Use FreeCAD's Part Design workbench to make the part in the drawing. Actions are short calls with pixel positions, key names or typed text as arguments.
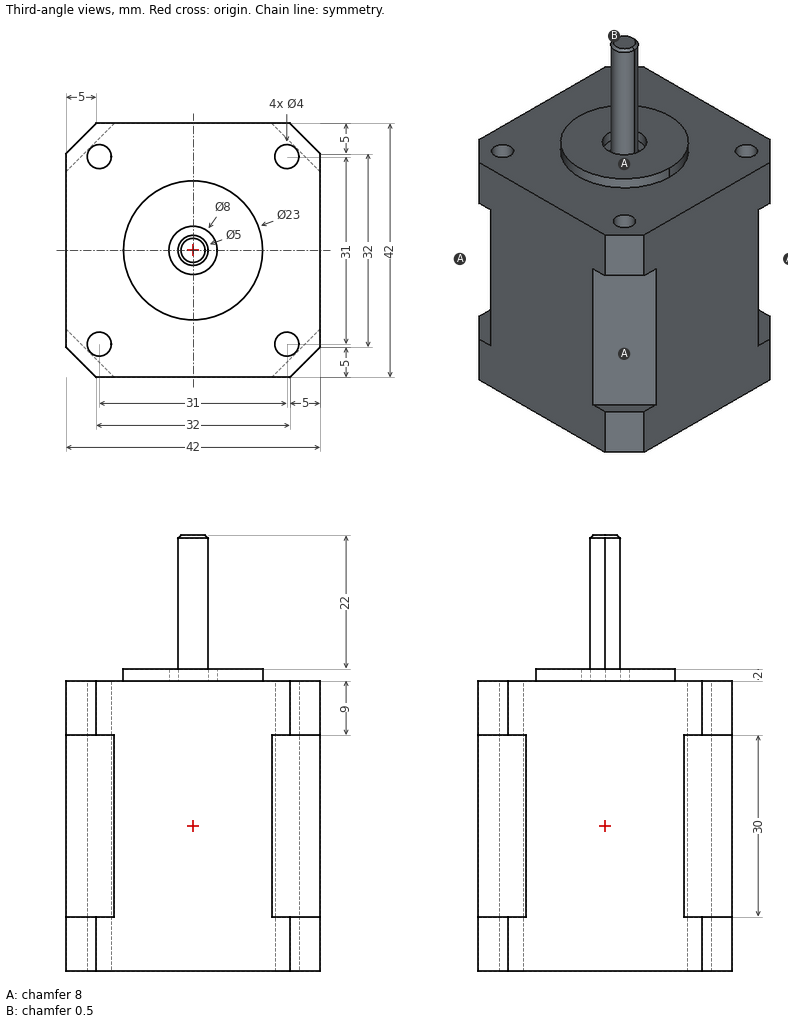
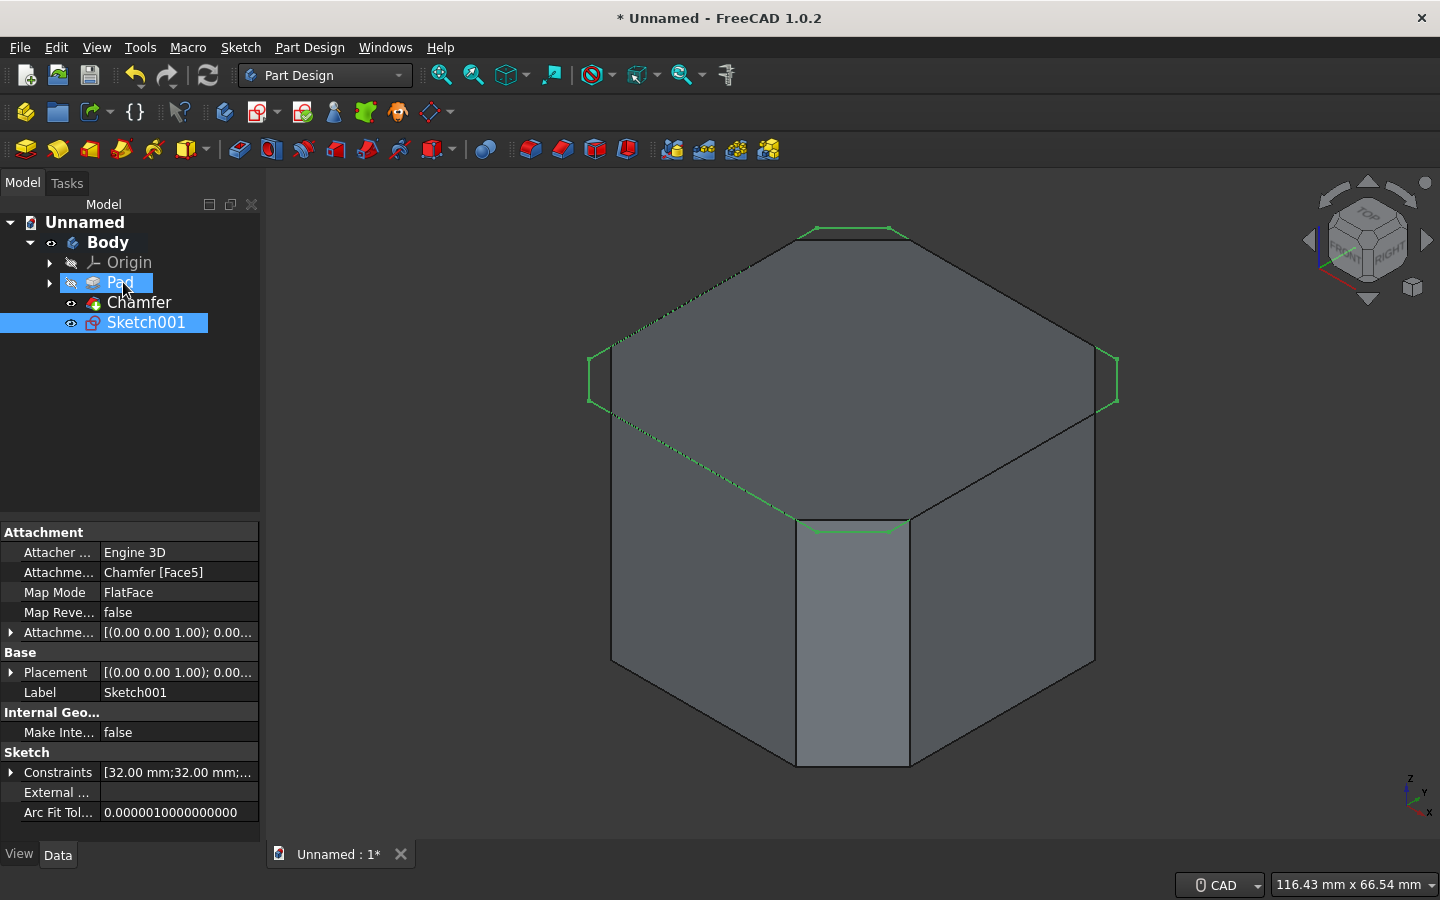
click(26, 150)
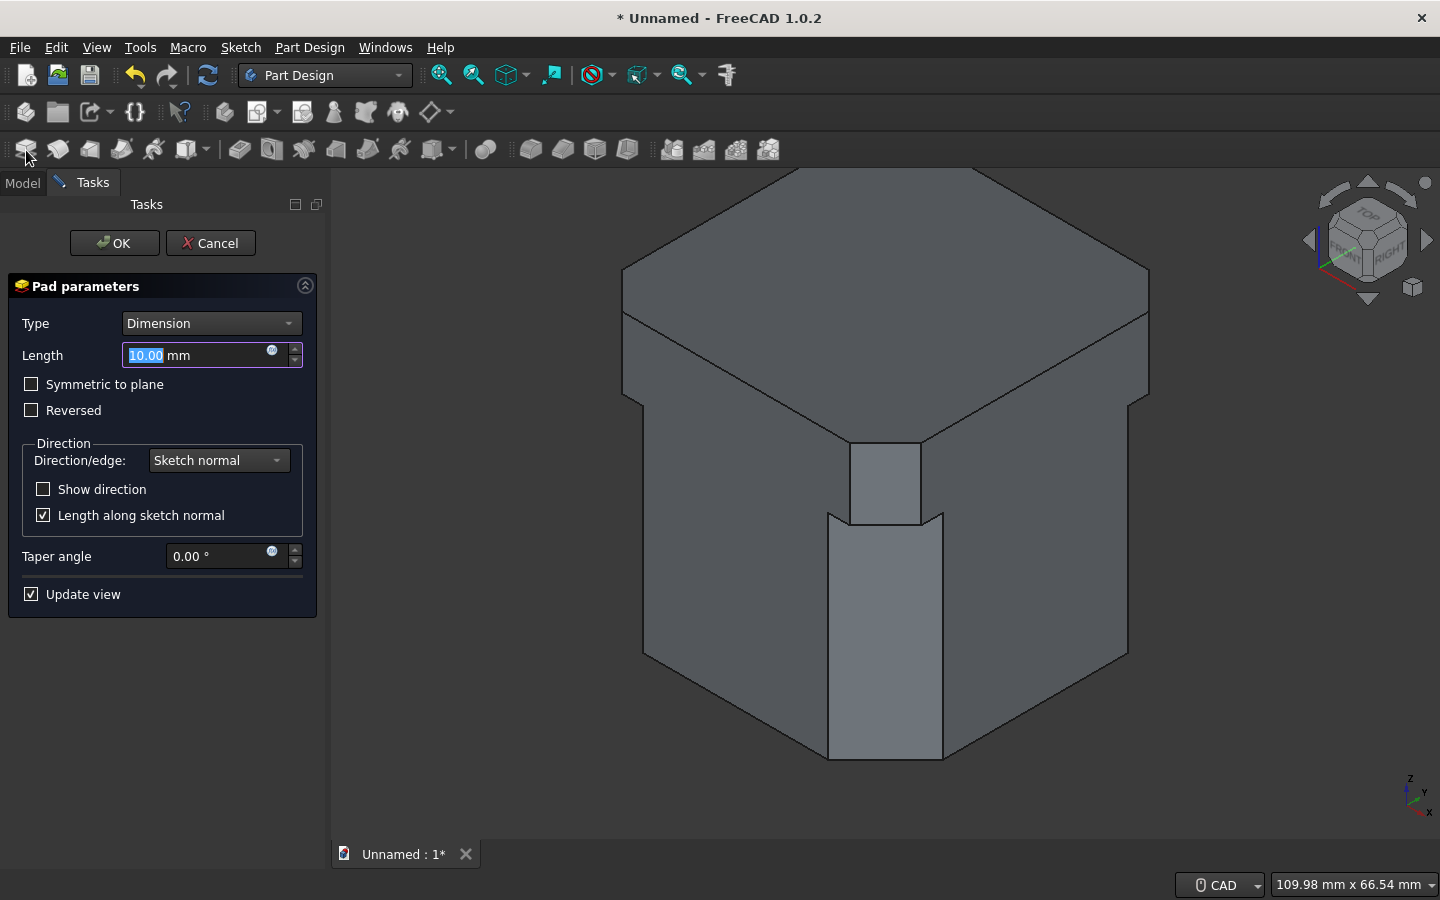
text(9)
key(Tab)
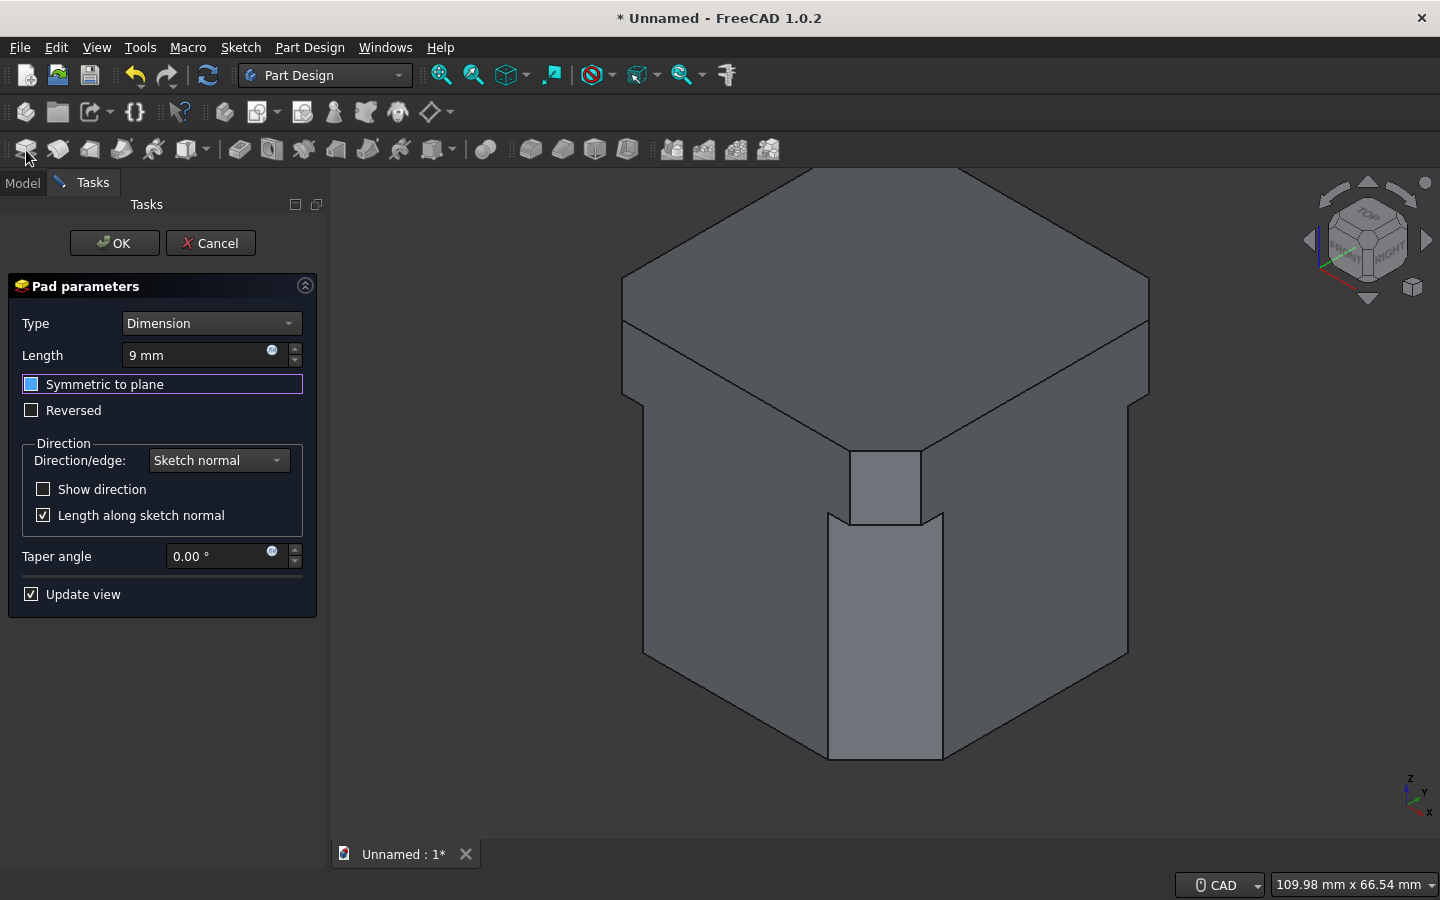
click(115, 243)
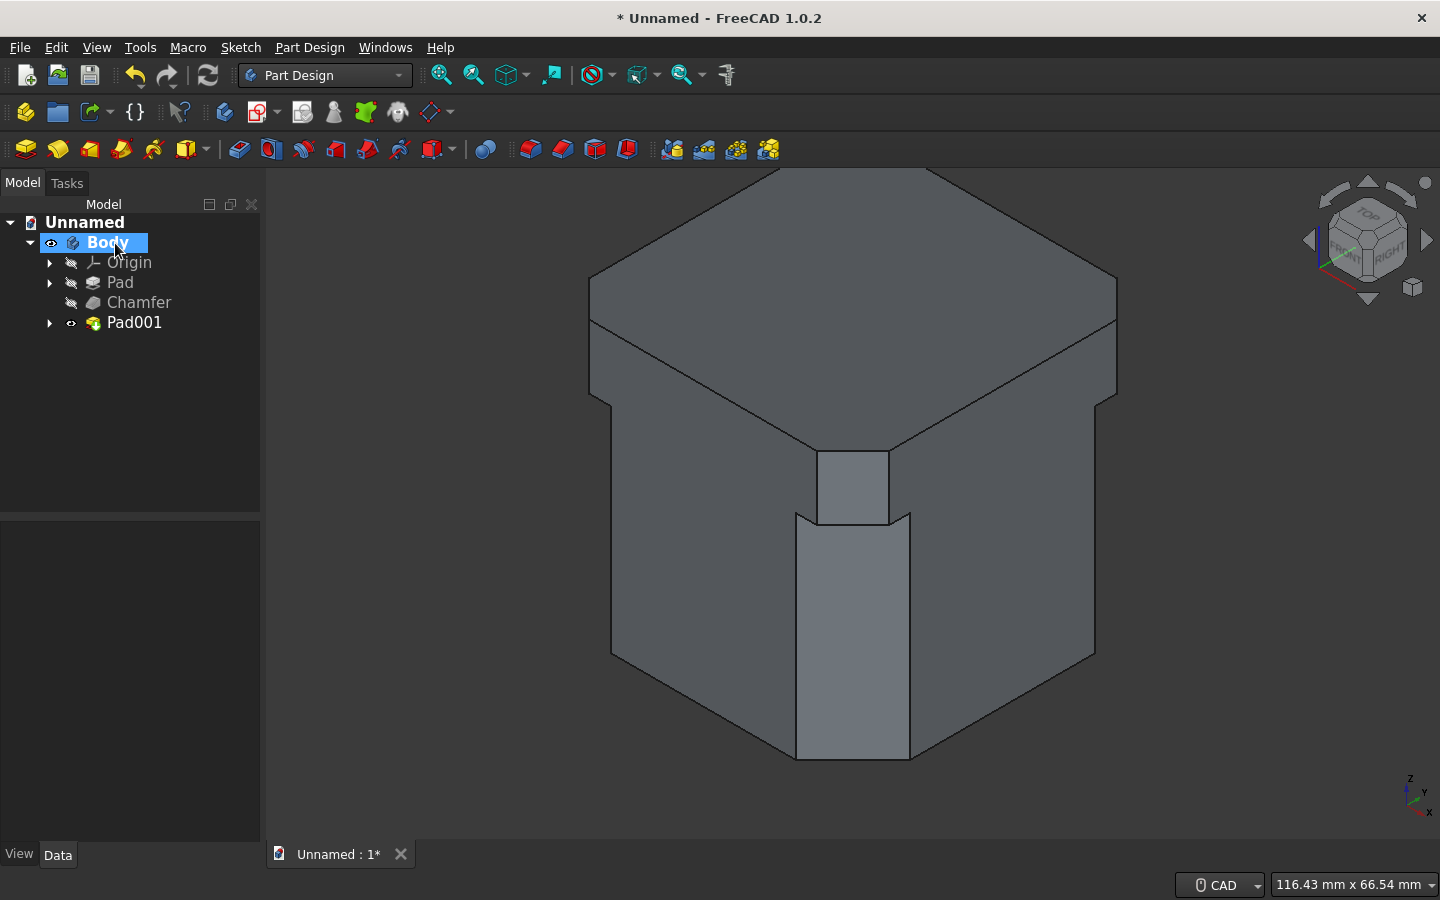
click(442, 76)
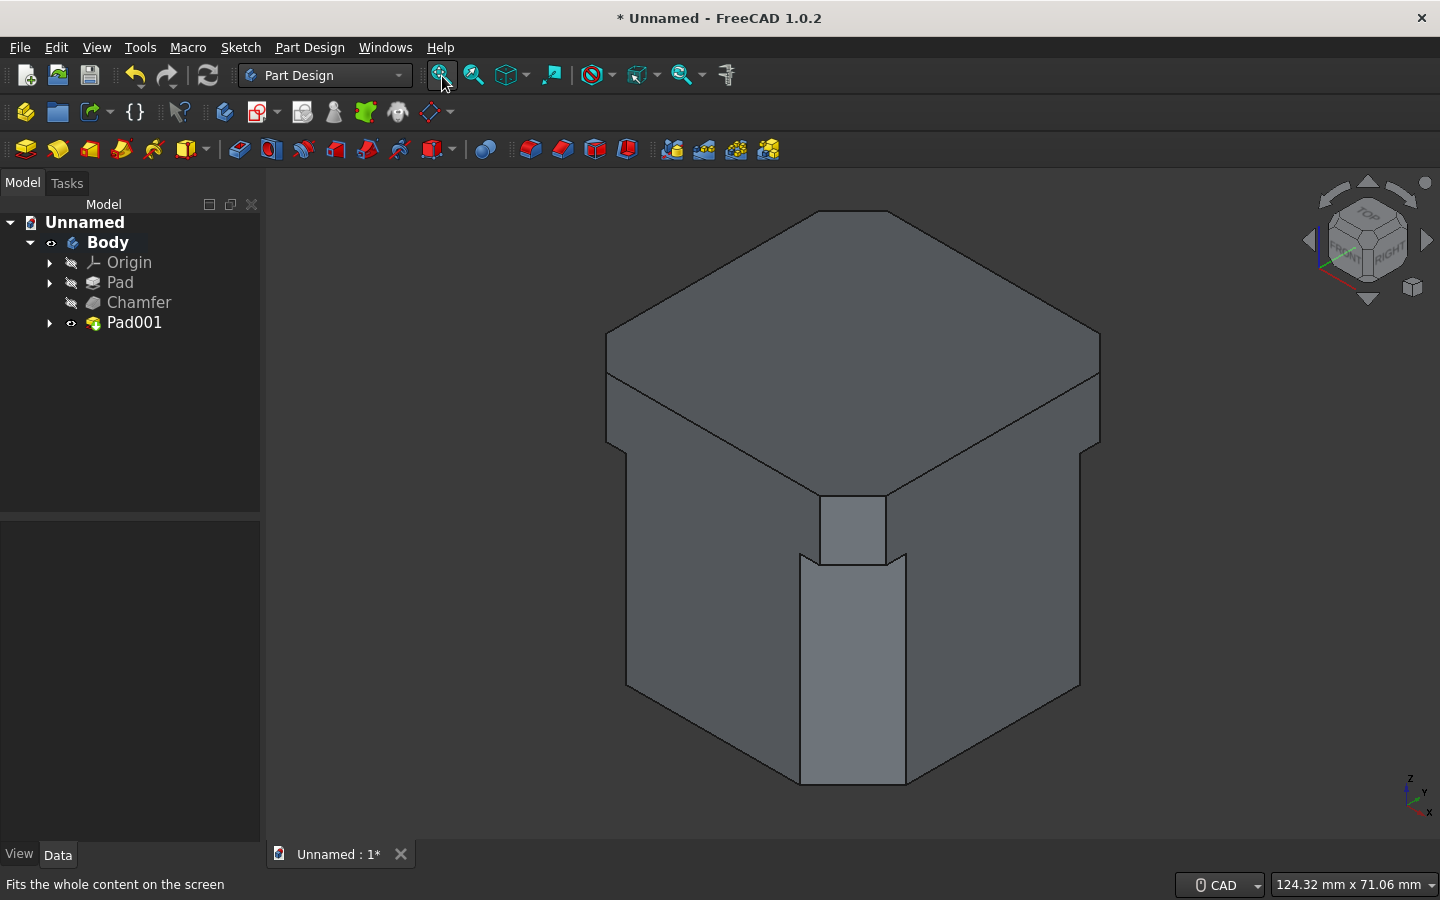
click(116, 323)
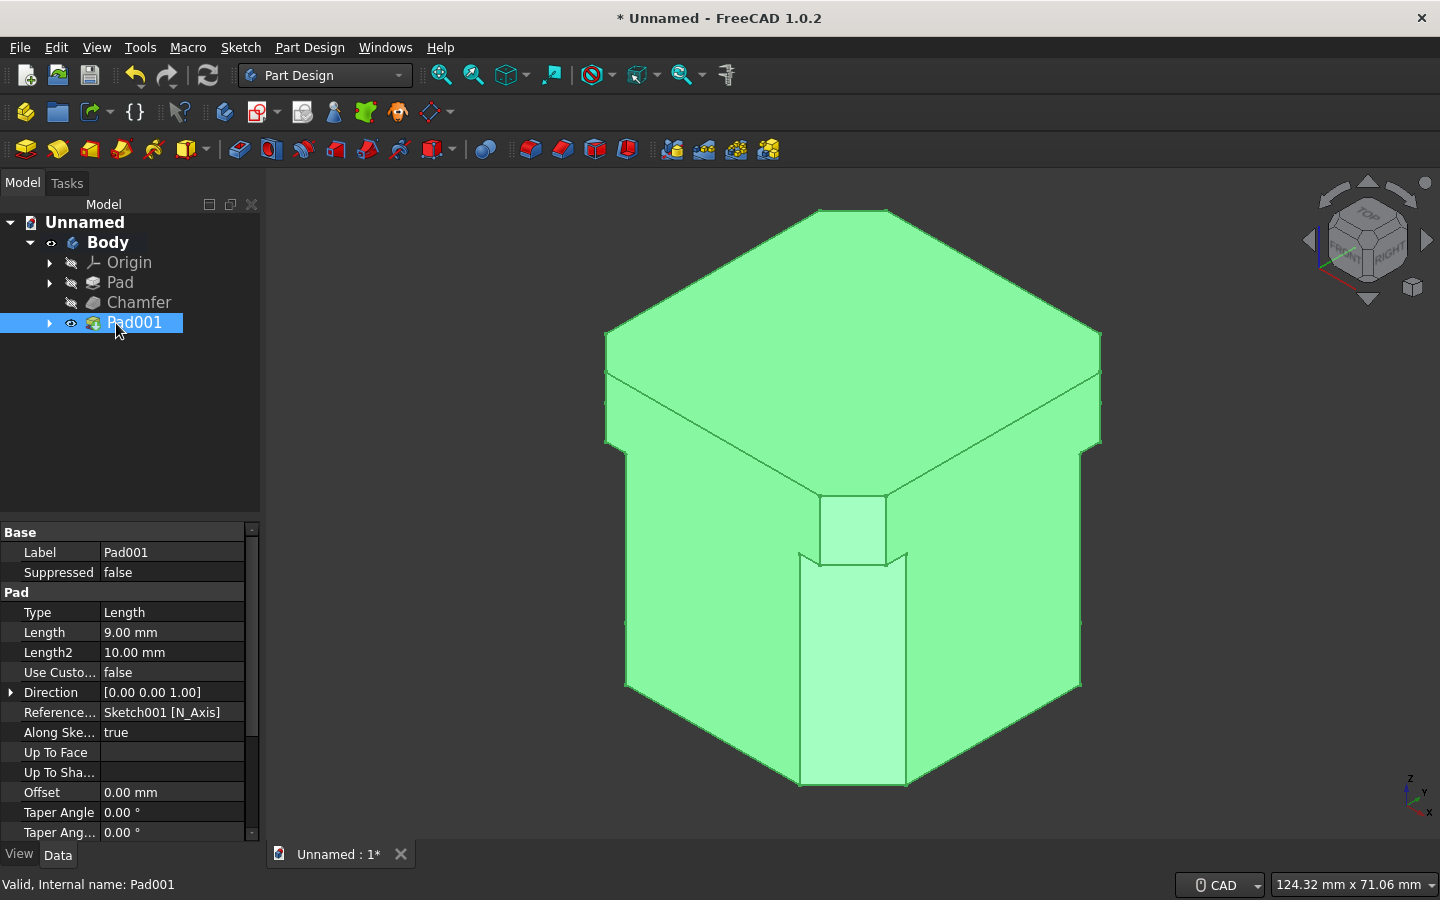
click(672, 150)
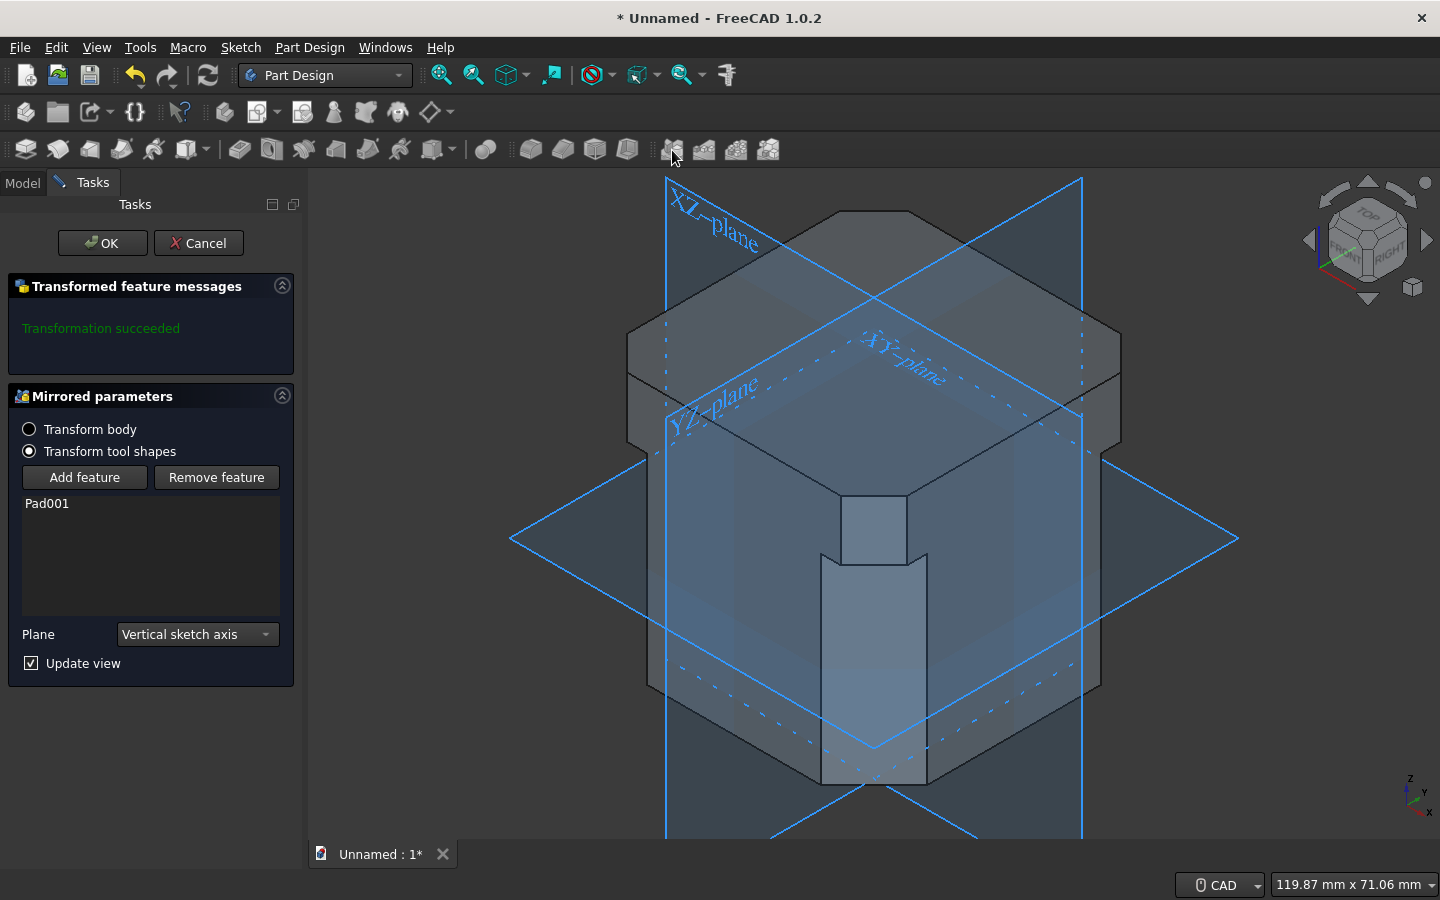
click(198, 634)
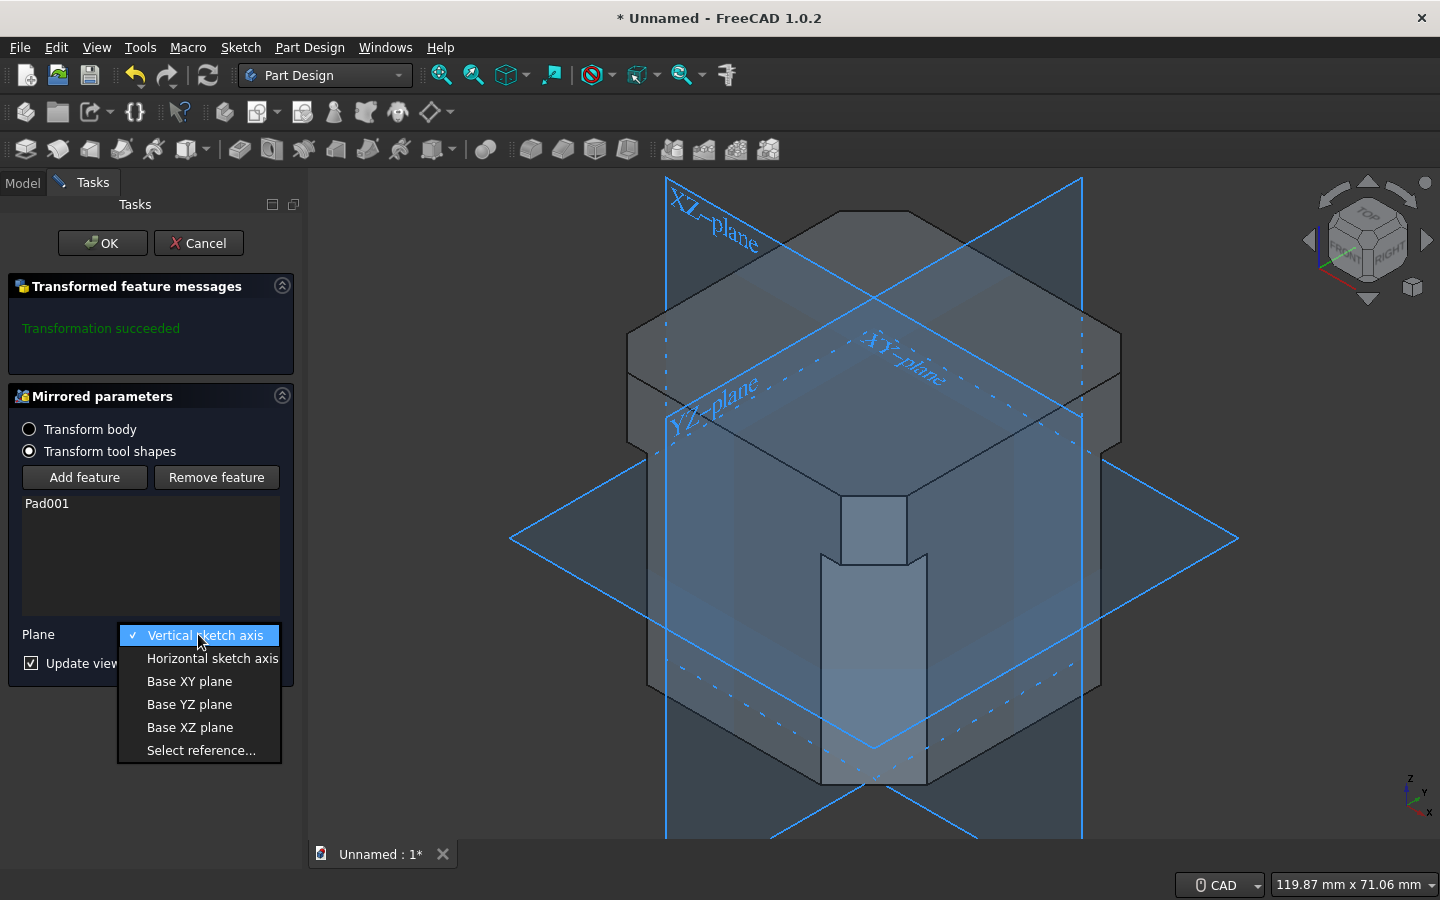
click(198, 682)